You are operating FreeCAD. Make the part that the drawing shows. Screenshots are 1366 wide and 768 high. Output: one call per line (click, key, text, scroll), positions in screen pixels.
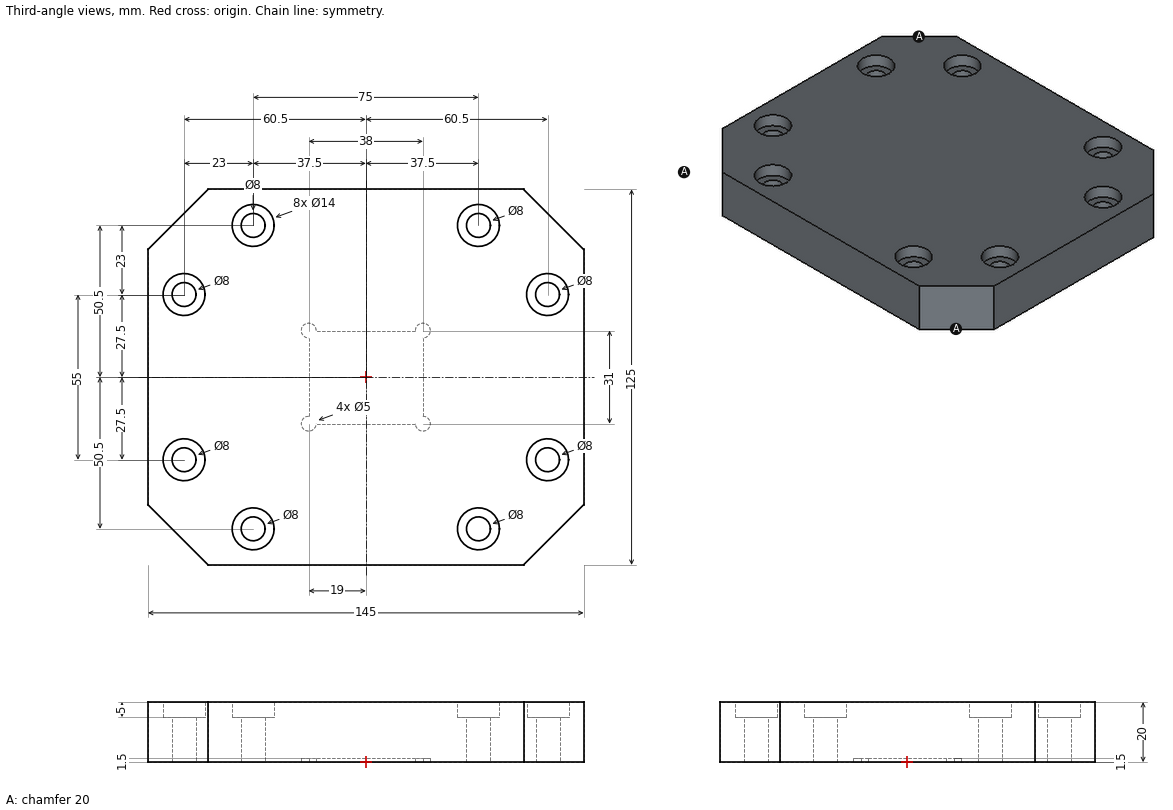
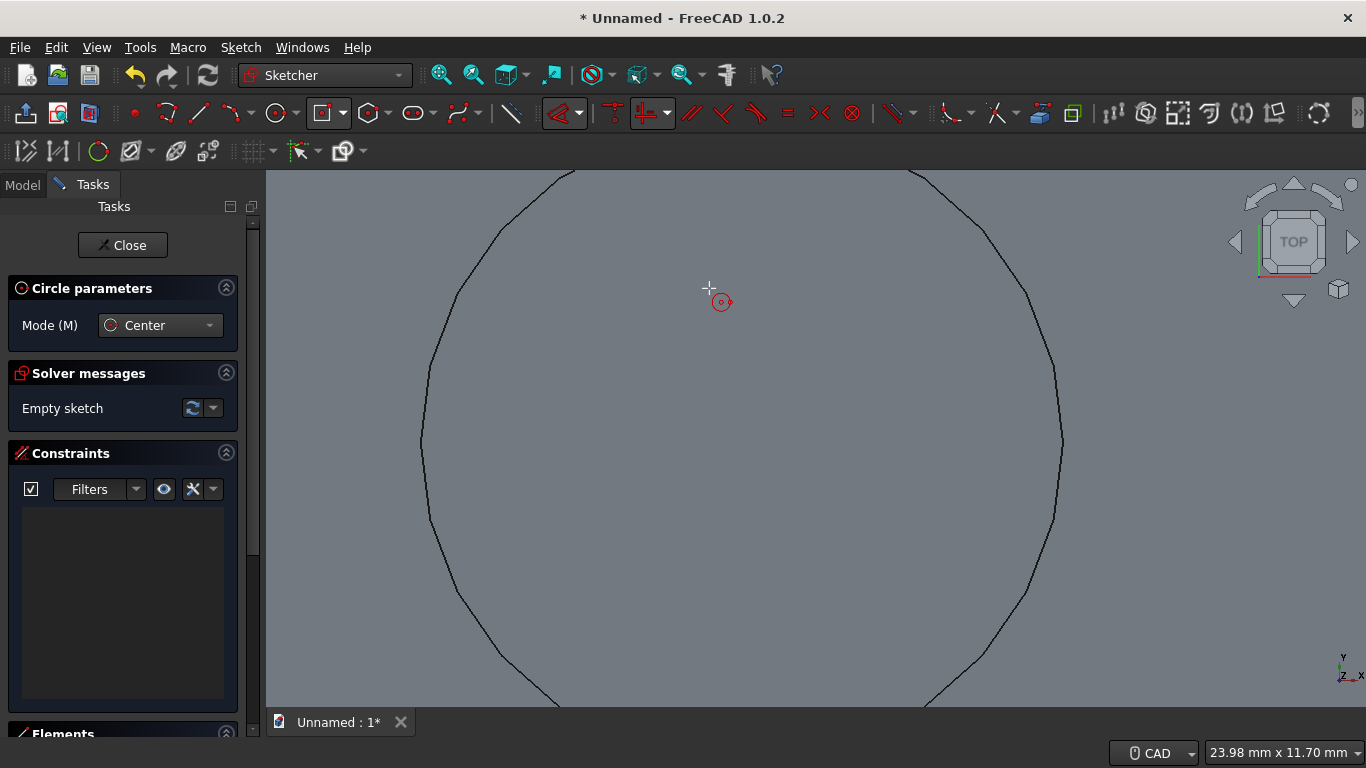
click(742, 443)
click(872, 313)
key(Escape)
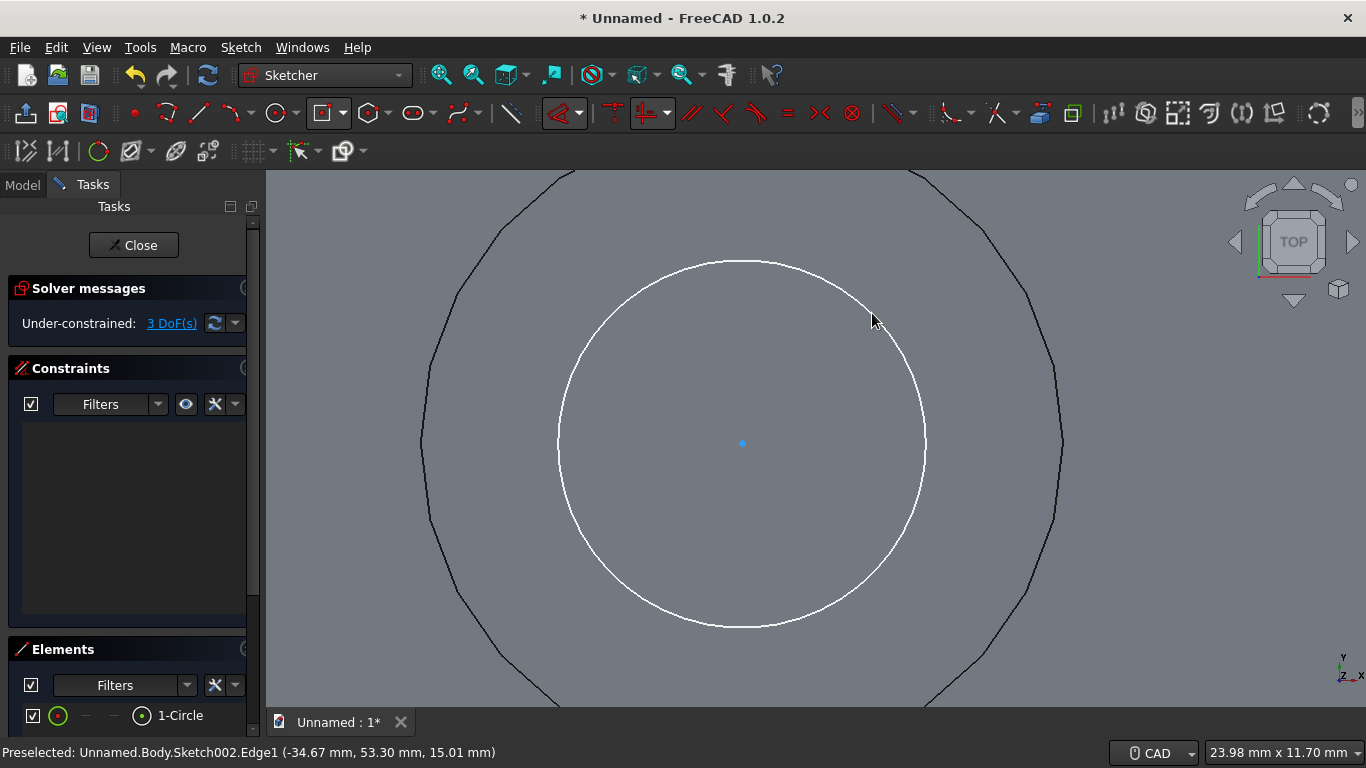
click(872, 314)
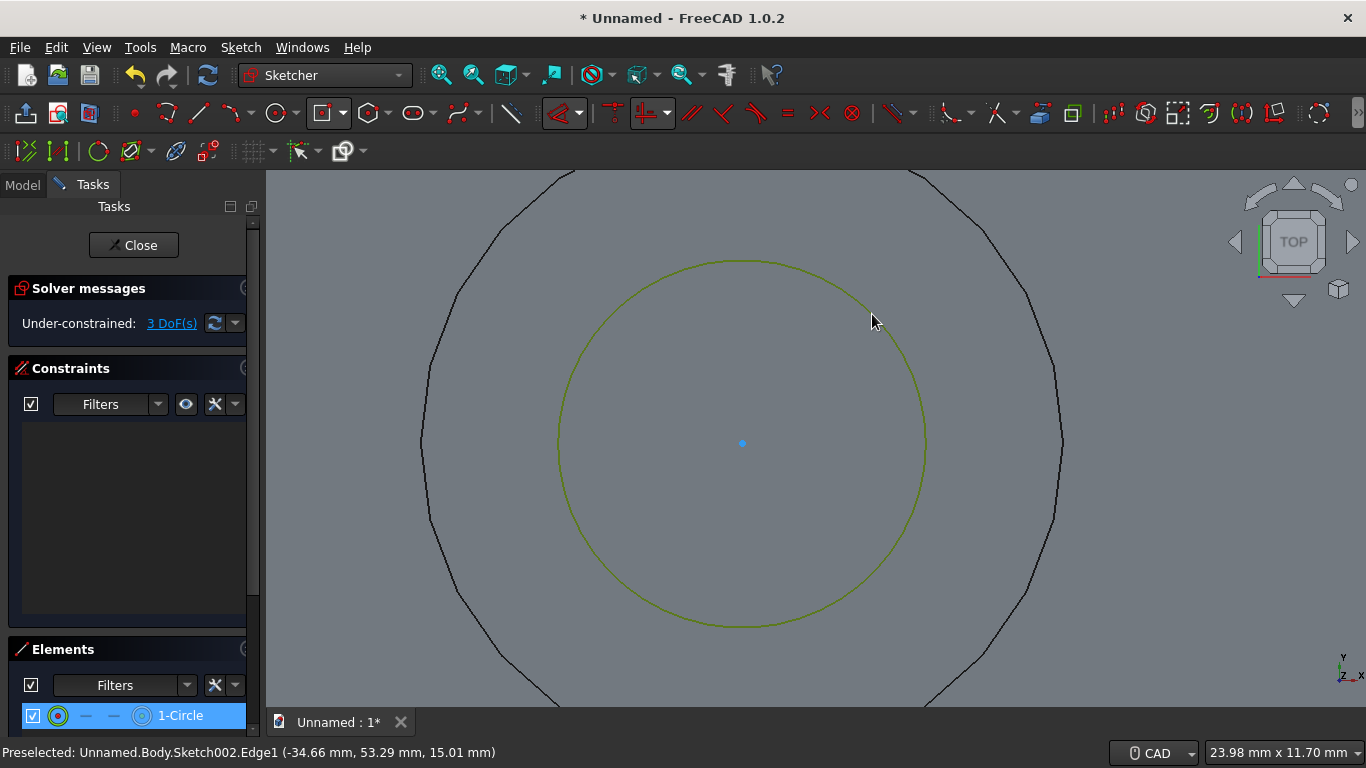
key(k)
key(o)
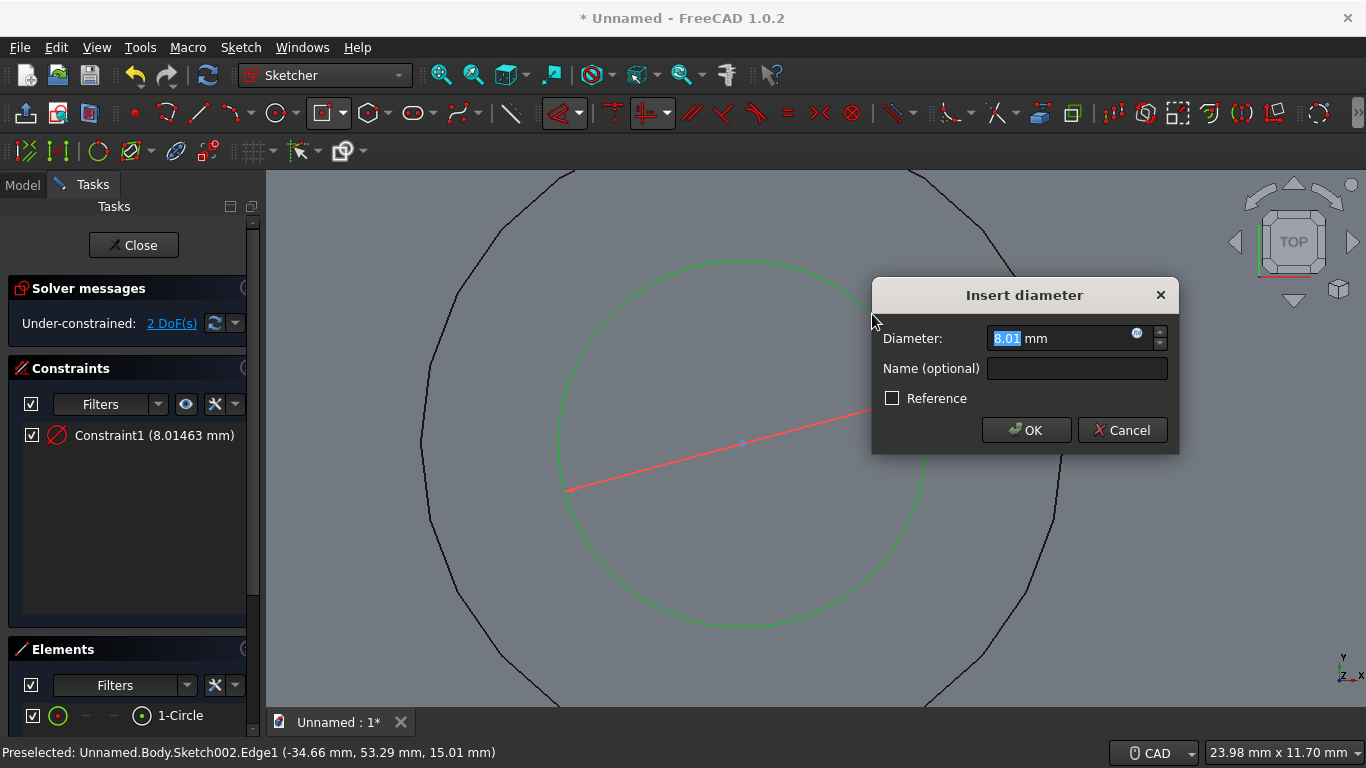
text(8)
key(Return)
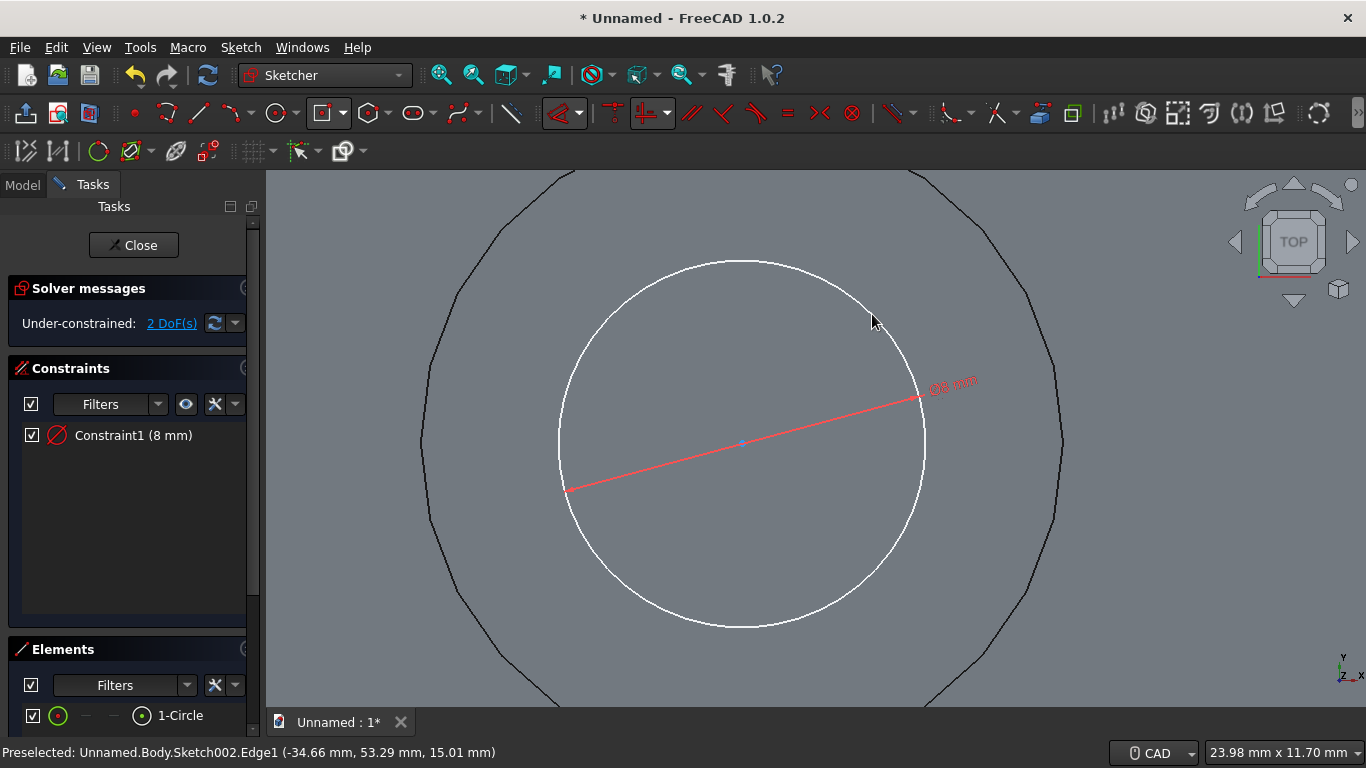
click(742, 444)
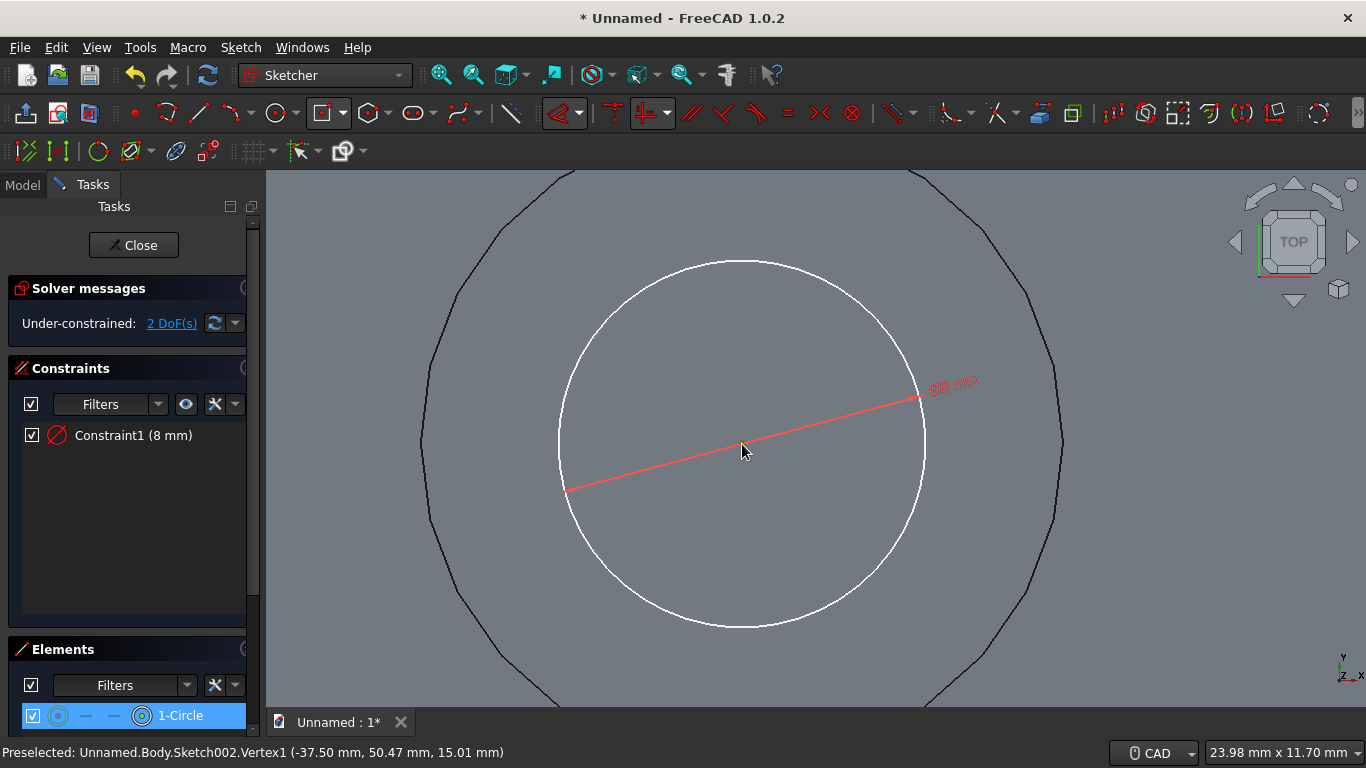
key(l)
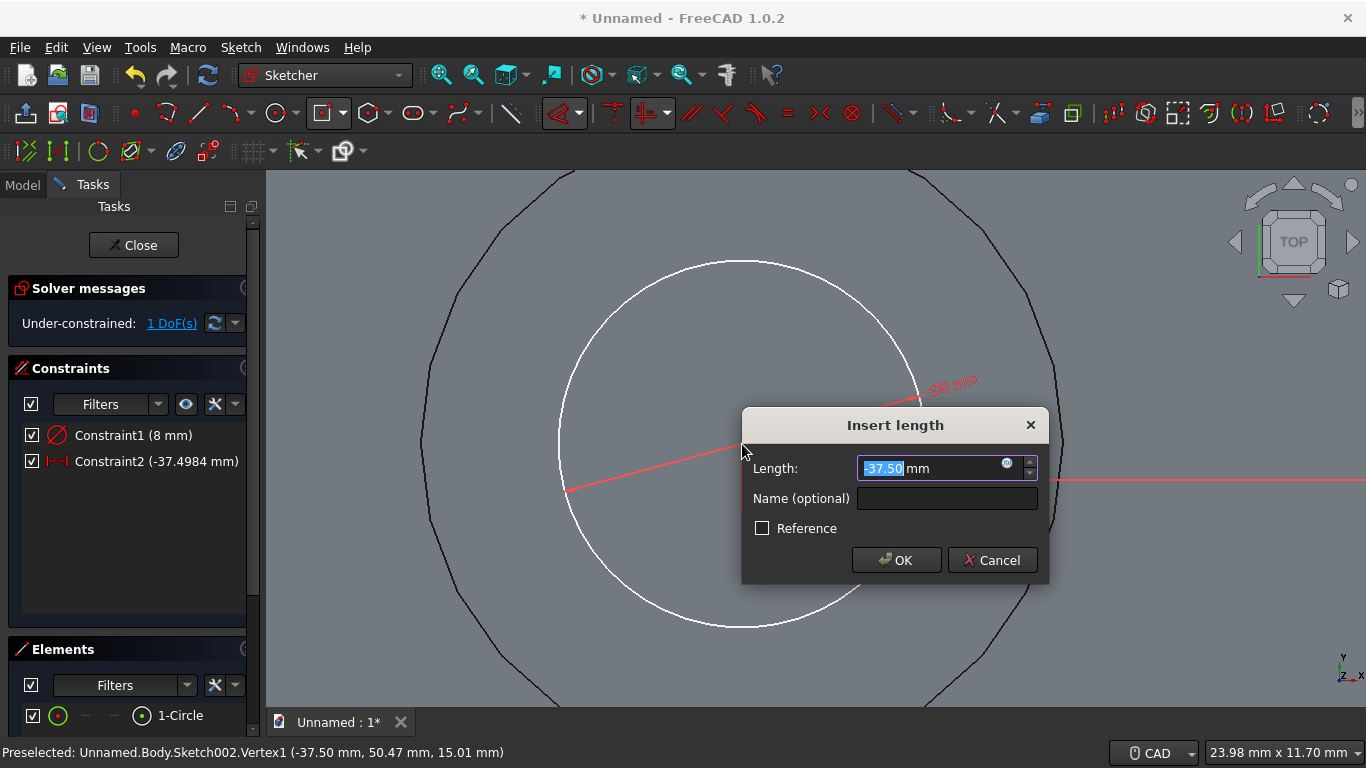
text(-37.5)
key(Return)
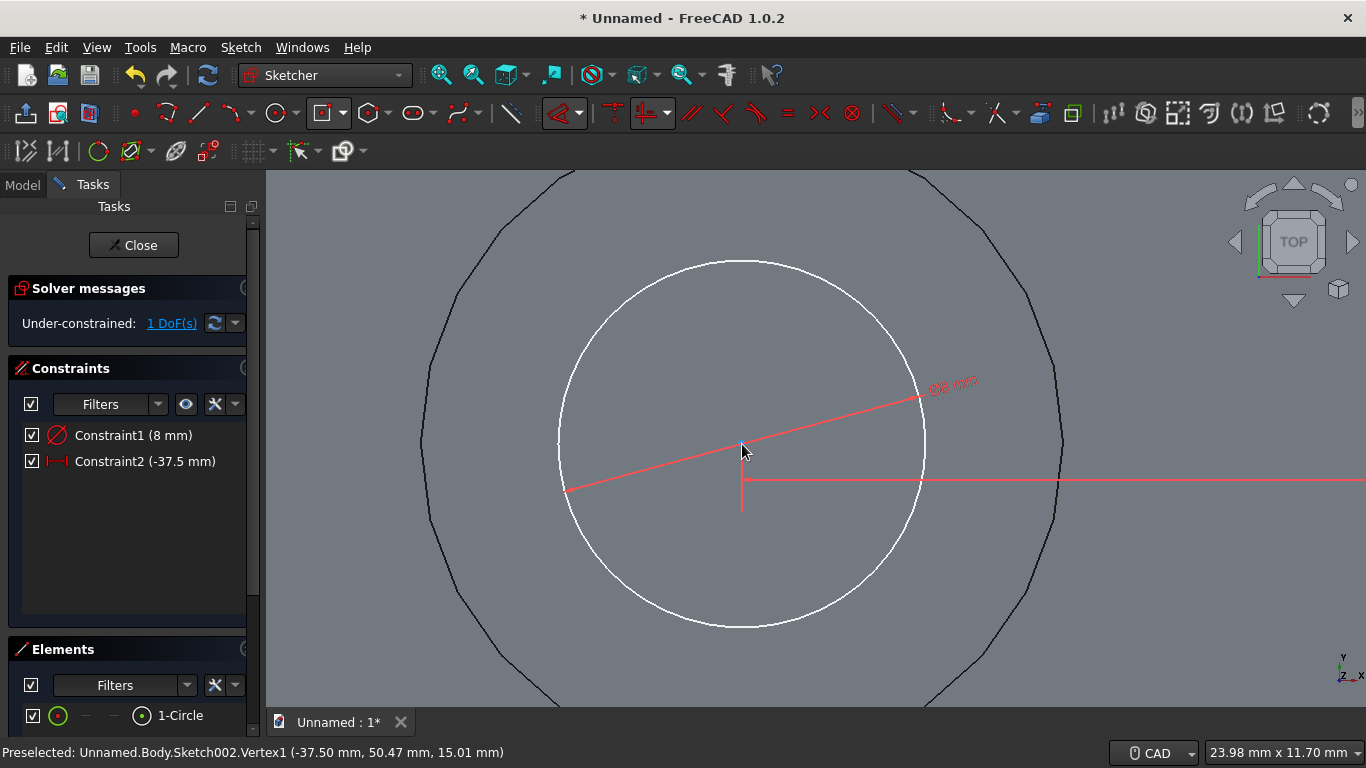
click(742, 444)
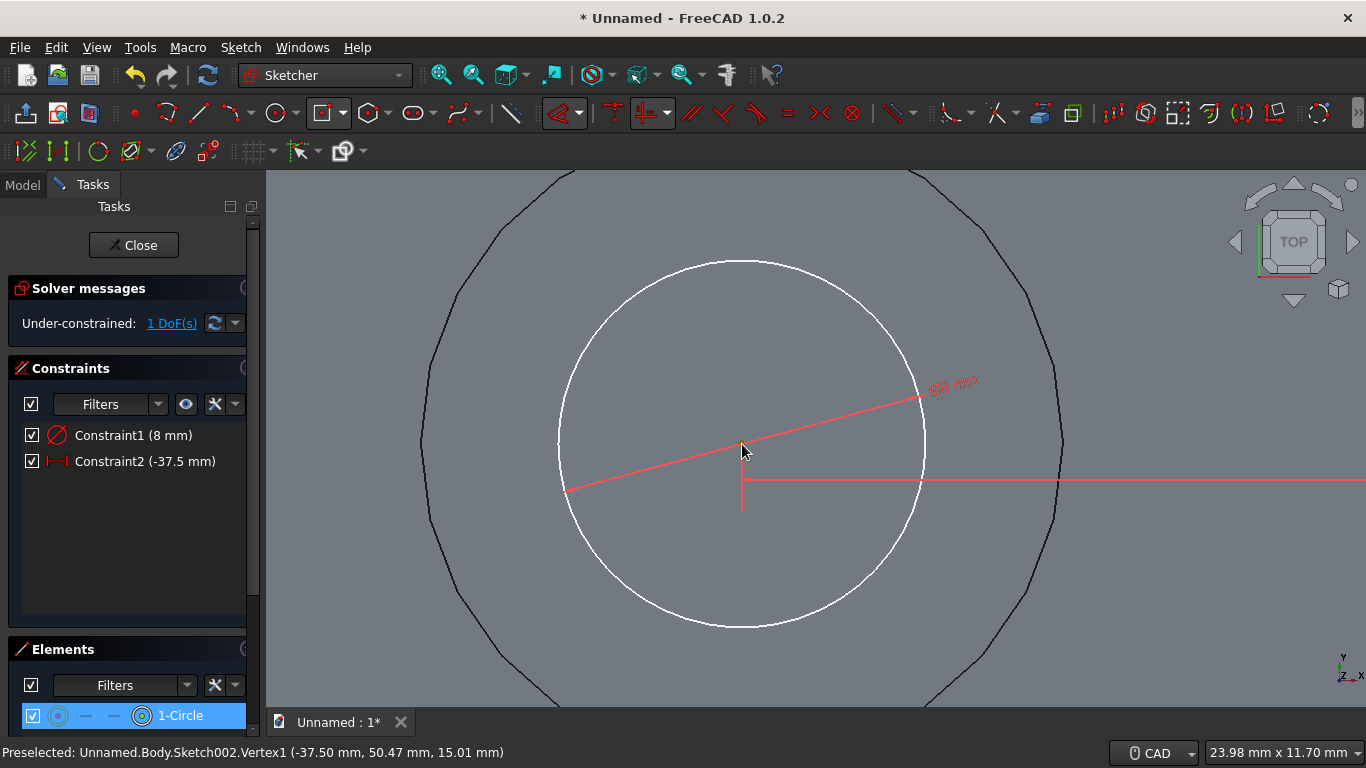
click(582, 114)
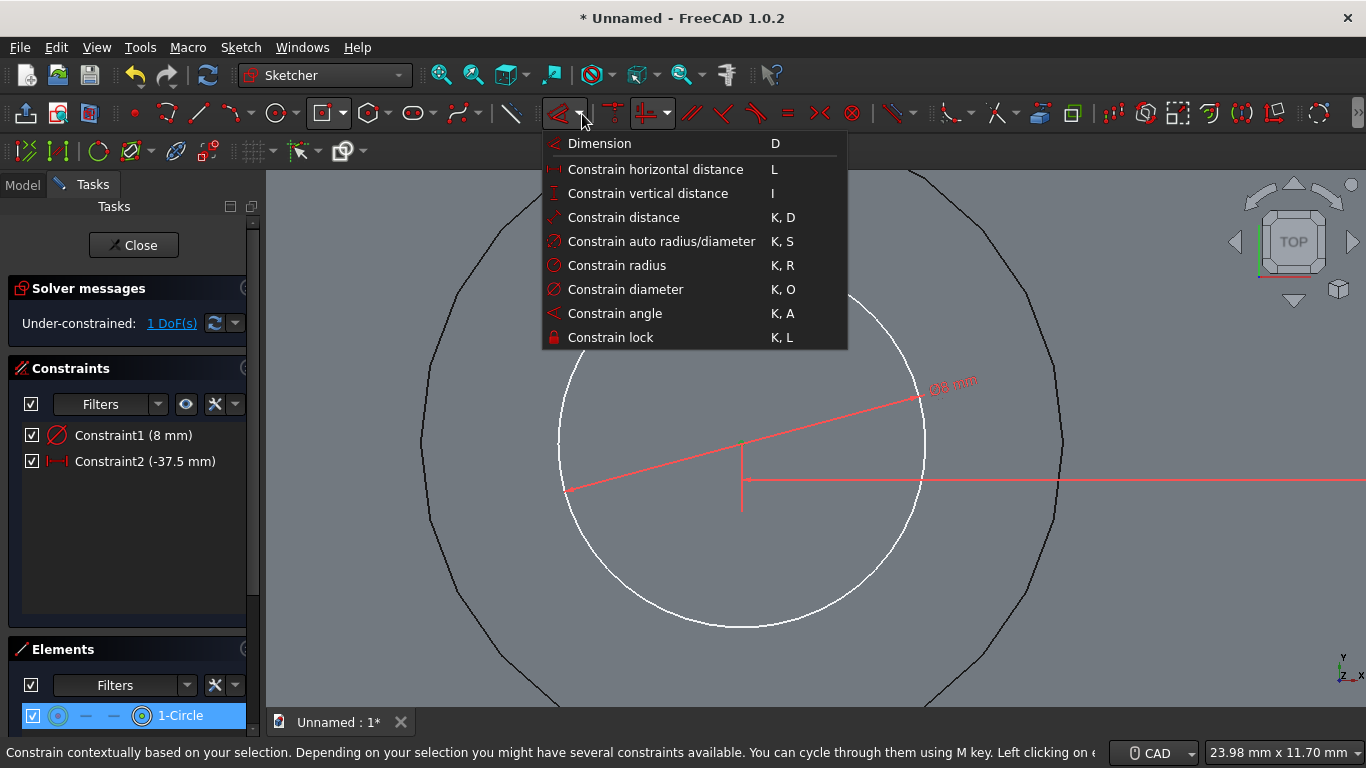
click(695, 193)